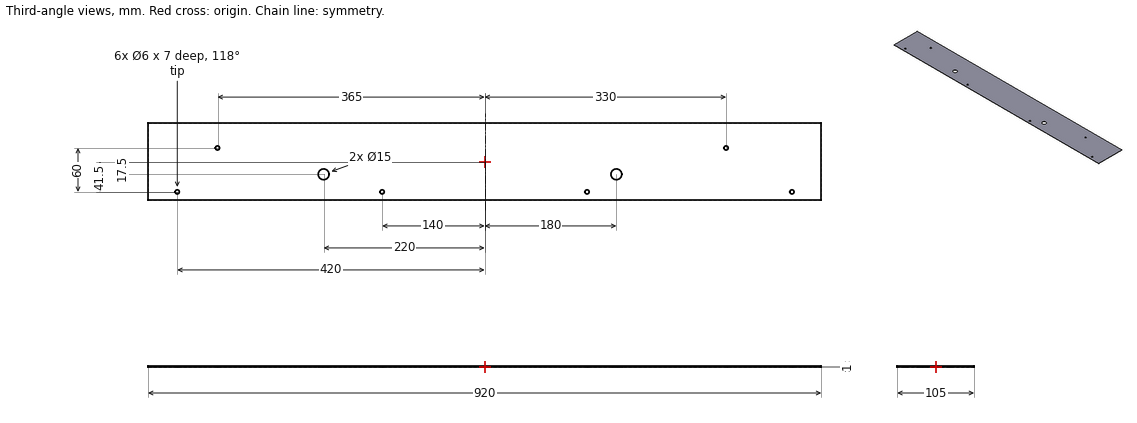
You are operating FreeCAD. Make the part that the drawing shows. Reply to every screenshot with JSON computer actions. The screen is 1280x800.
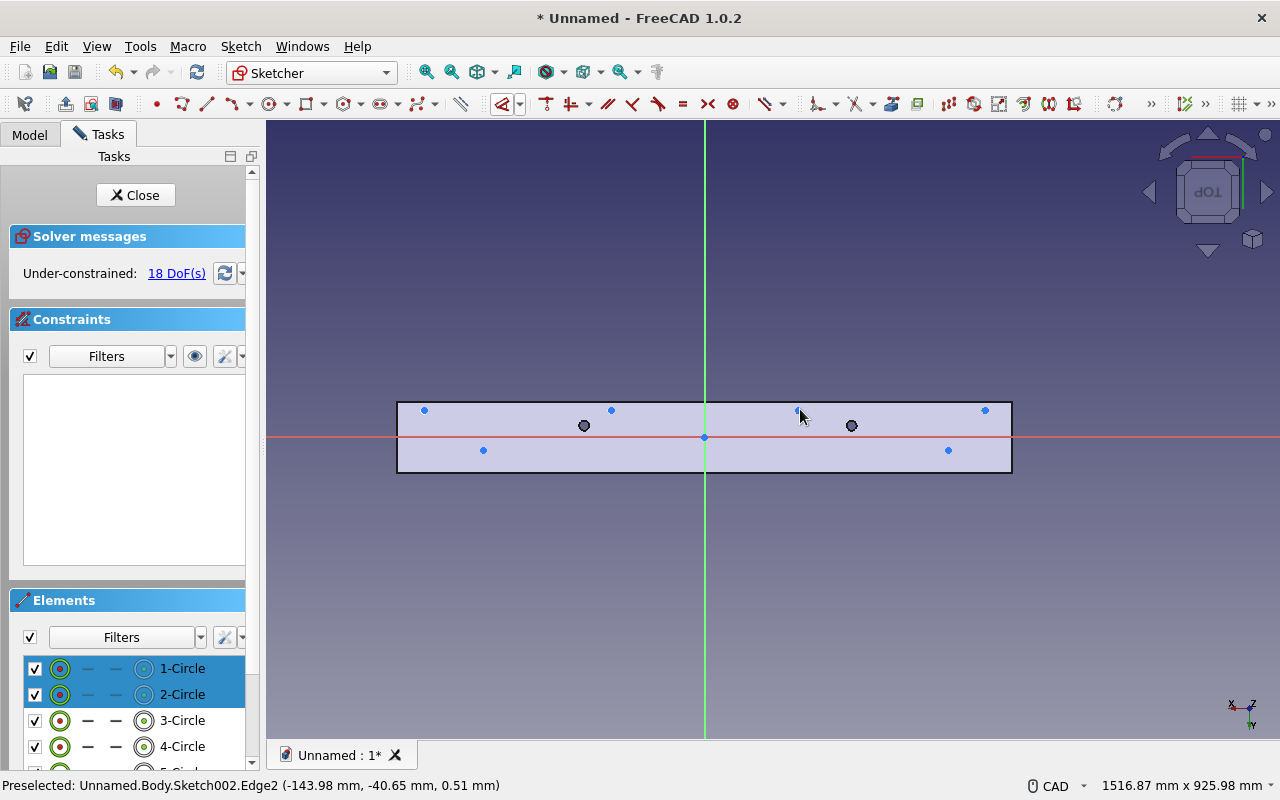
{"action": "scroll", "coordinate": [613, 409], "scroll_direction": "up", "scroll_amount": 9}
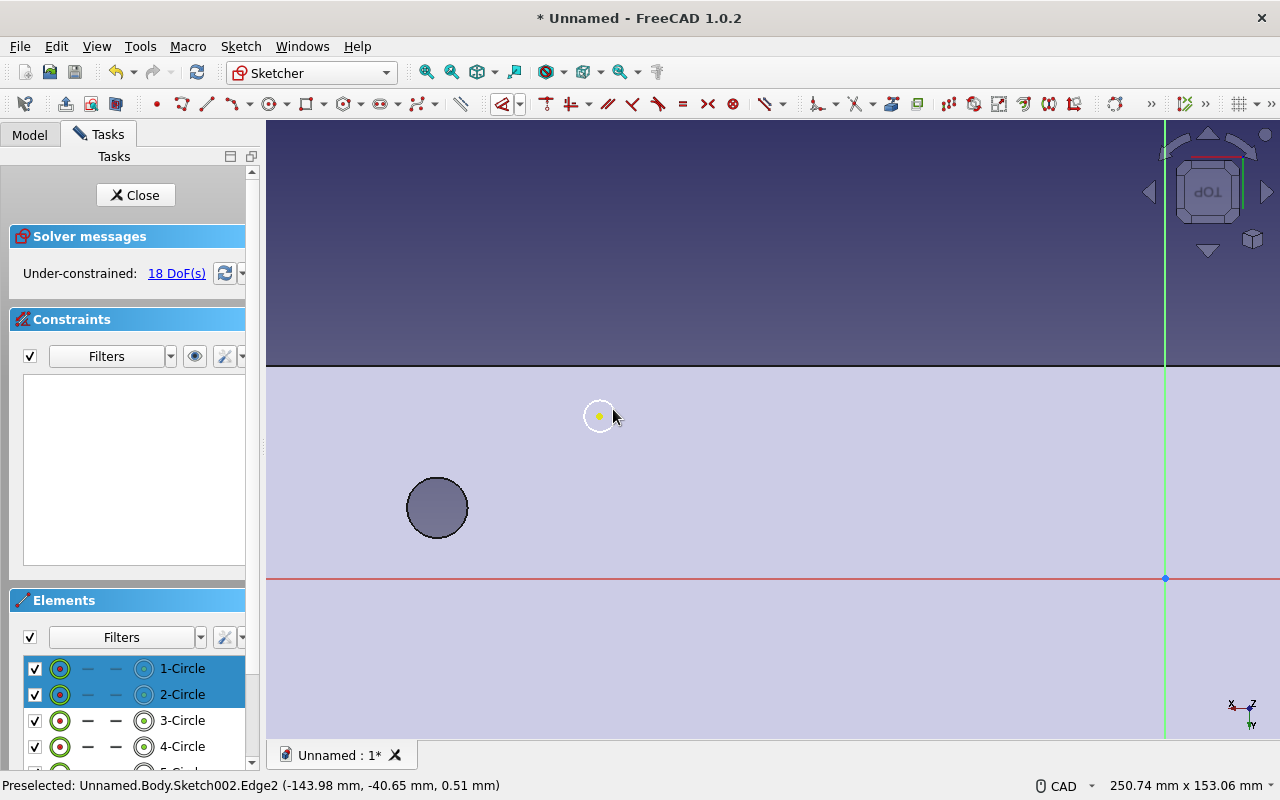
{"action": "left_click", "coordinate": [611, 405]}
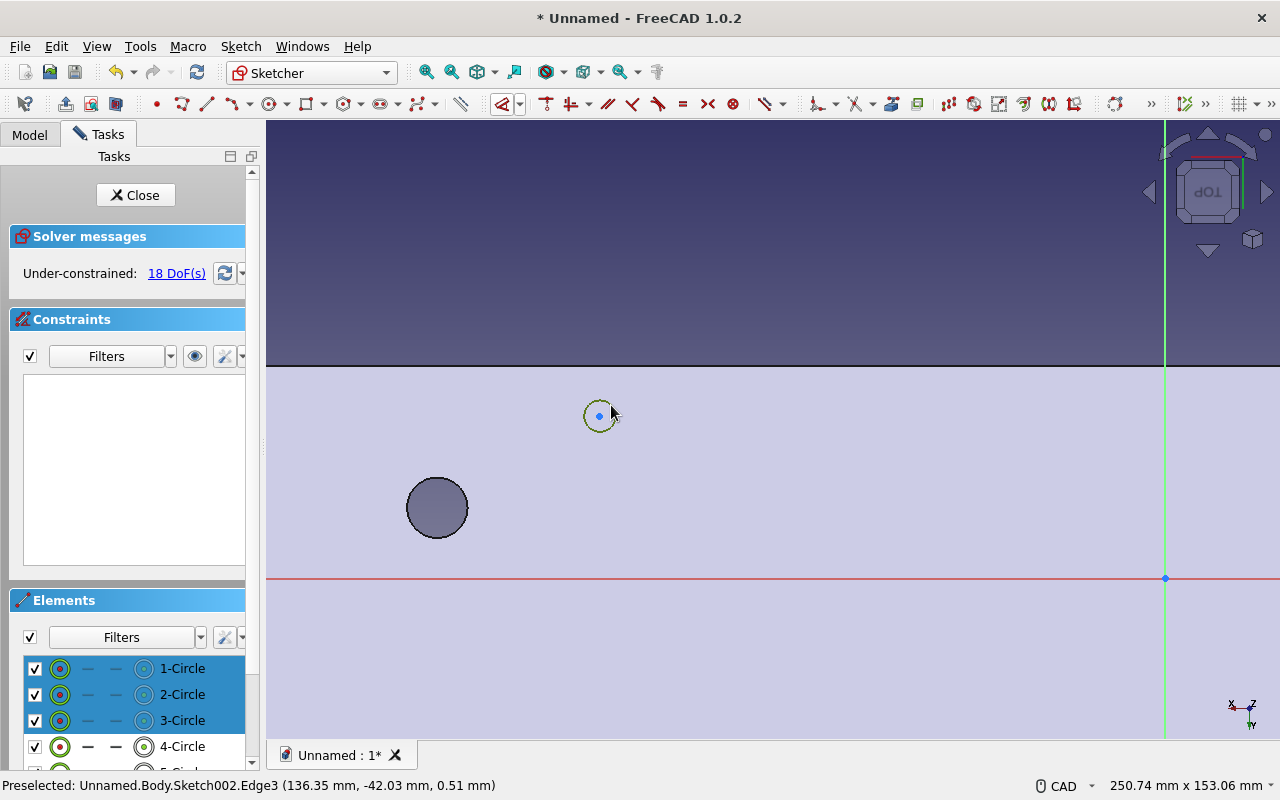
{"action": "scroll", "coordinate": [613, 409], "scroll_direction": "down", "scroll_amount": 9}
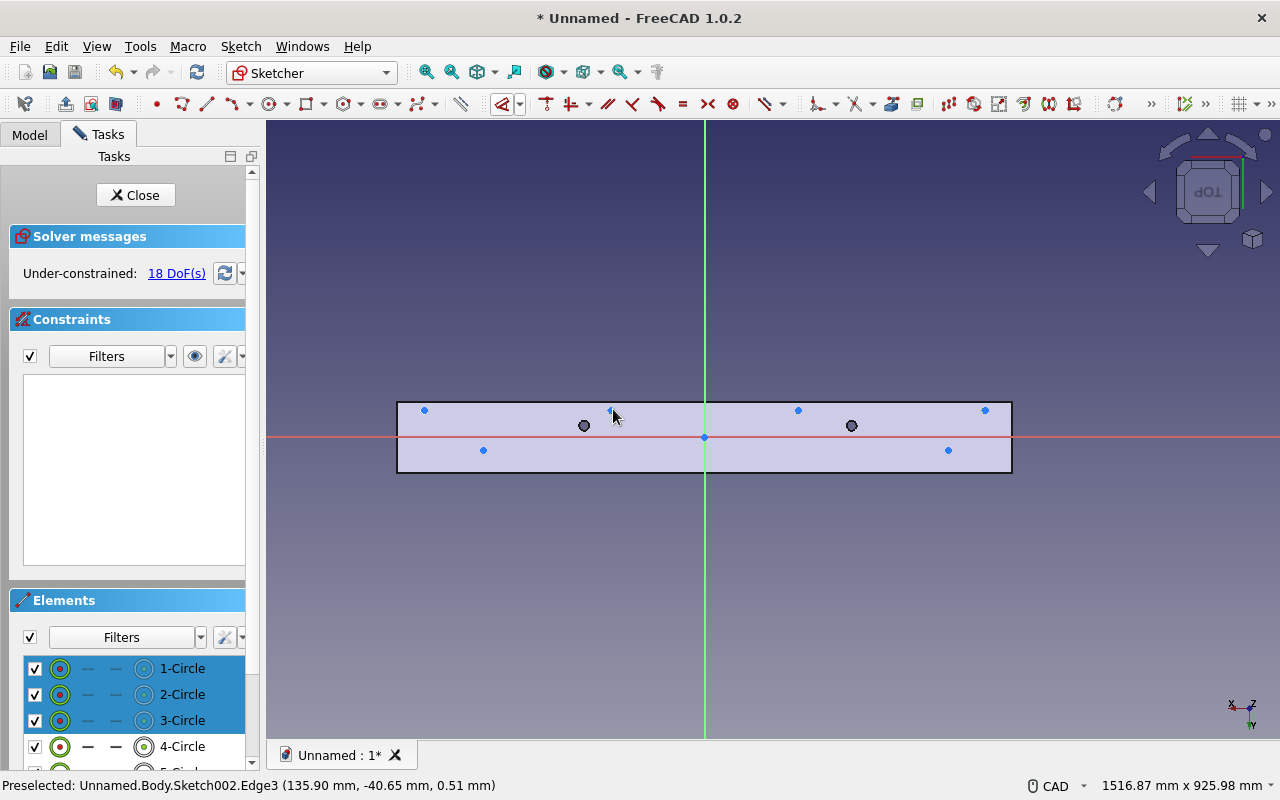
{"action": "scroll", "coordinate": [950, 449], "scroll_direction": "up", "scroll_amount": 9}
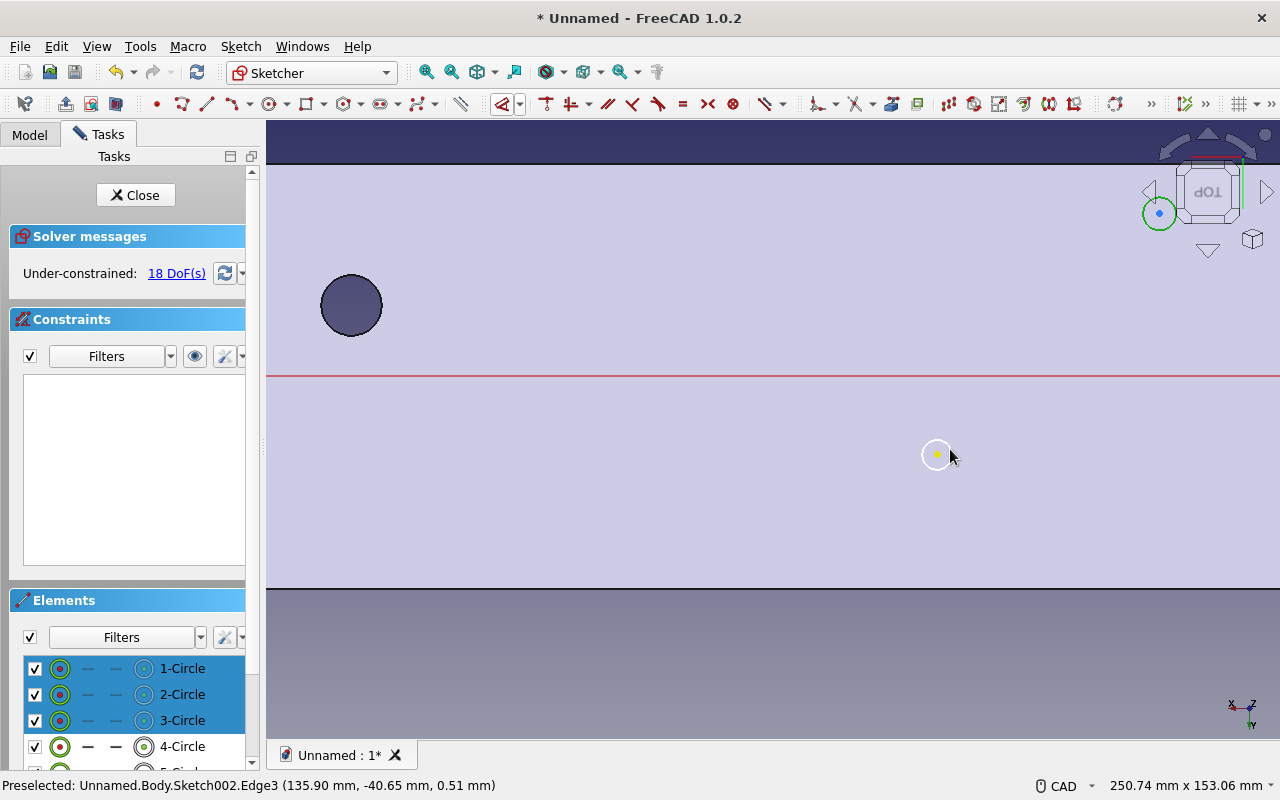
{"action": "left_click", "coordinate": [948, 444]}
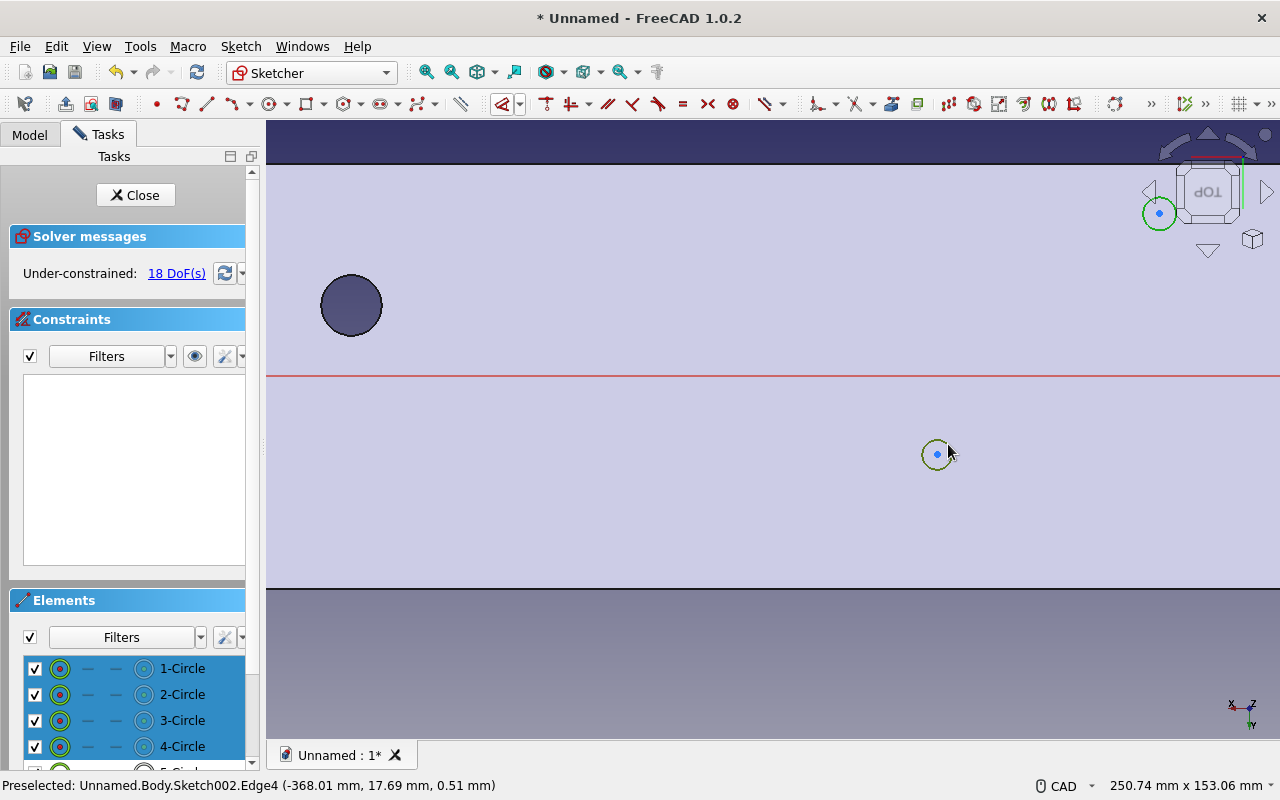
{"action": "scroll", "coordinate": [951, 449], "scroll_direction": "down", "scroll_amount": 9}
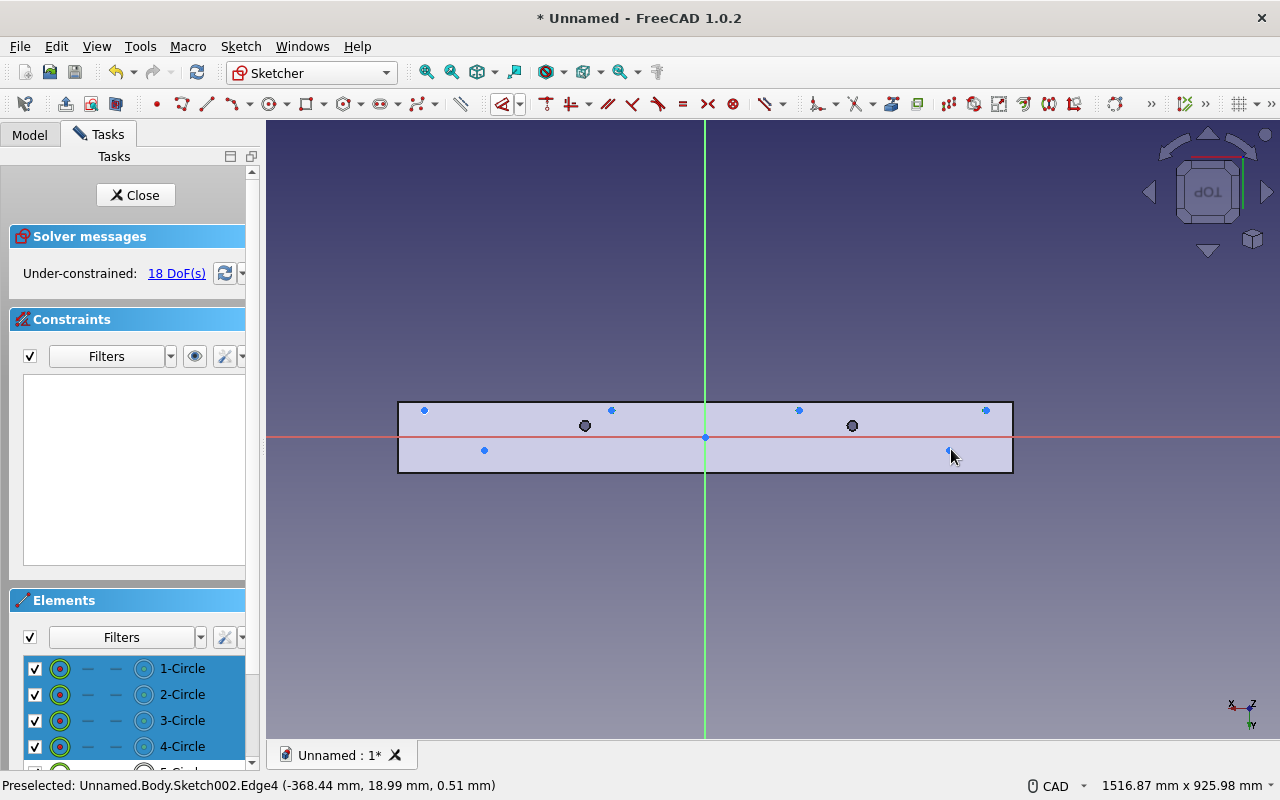
{"action": "scroll", "coordinate": [486, 449], "scroll_direction": "up", "scroll_amount": 9}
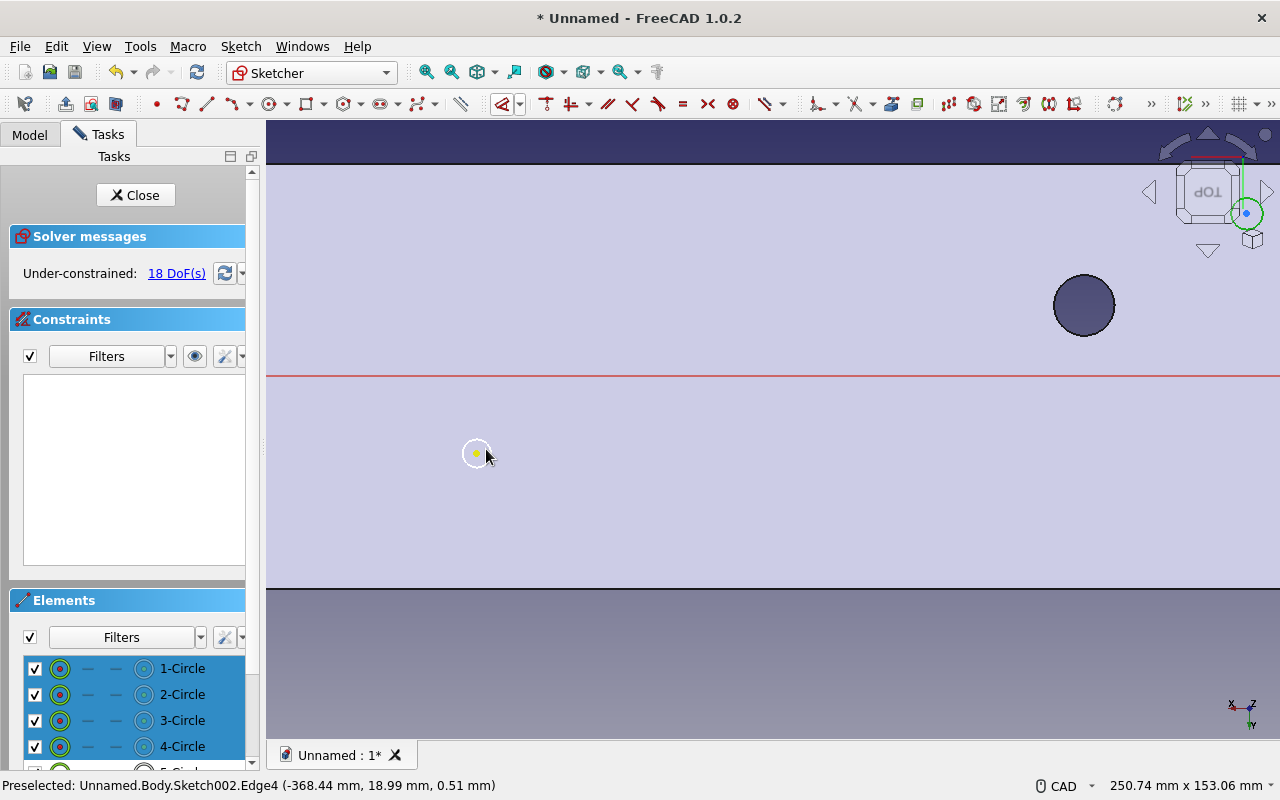
{"action": "left_click", "coordinate": [487, 444]}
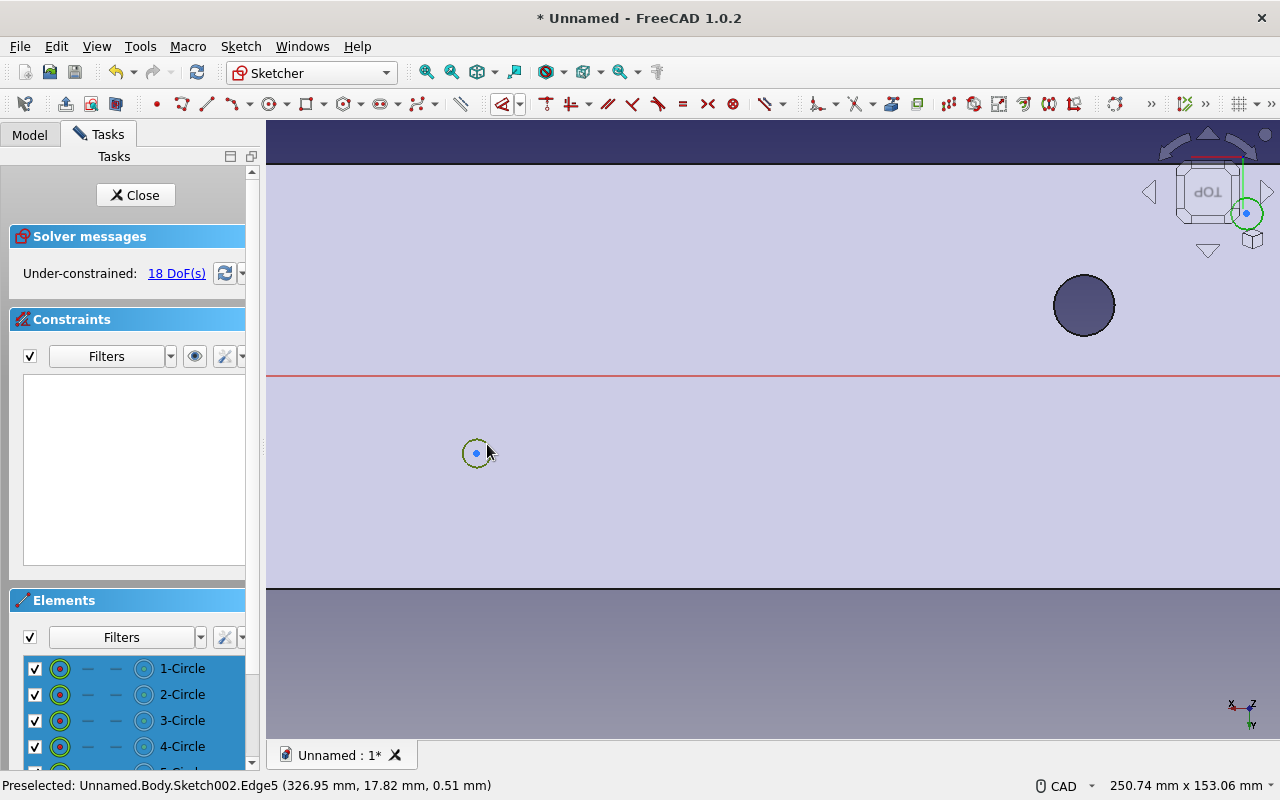
{"action": "scroll", "coordinate": [485, 449], "scroll_direction": "down", "scroll_amount": 9}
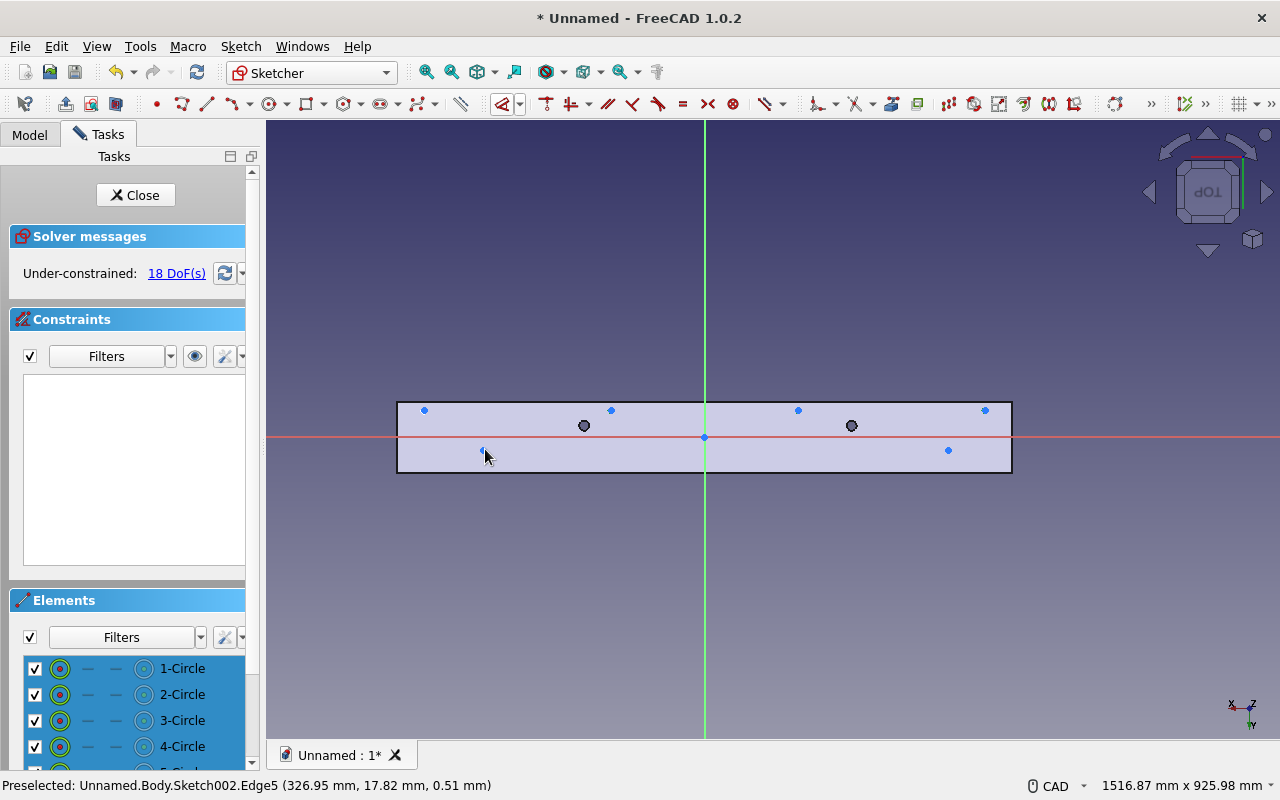
{"action": "scroll", "coordinate": [426, 409], "scroll_direction": "up", "scroll_amount": 8}